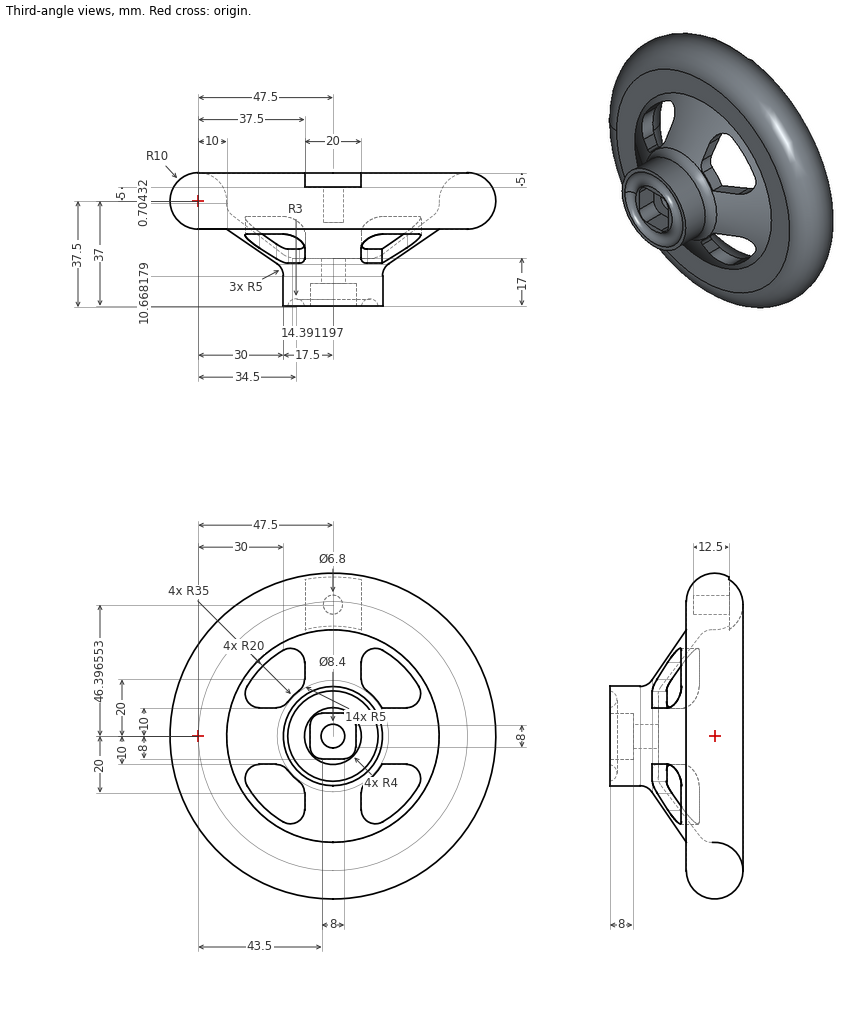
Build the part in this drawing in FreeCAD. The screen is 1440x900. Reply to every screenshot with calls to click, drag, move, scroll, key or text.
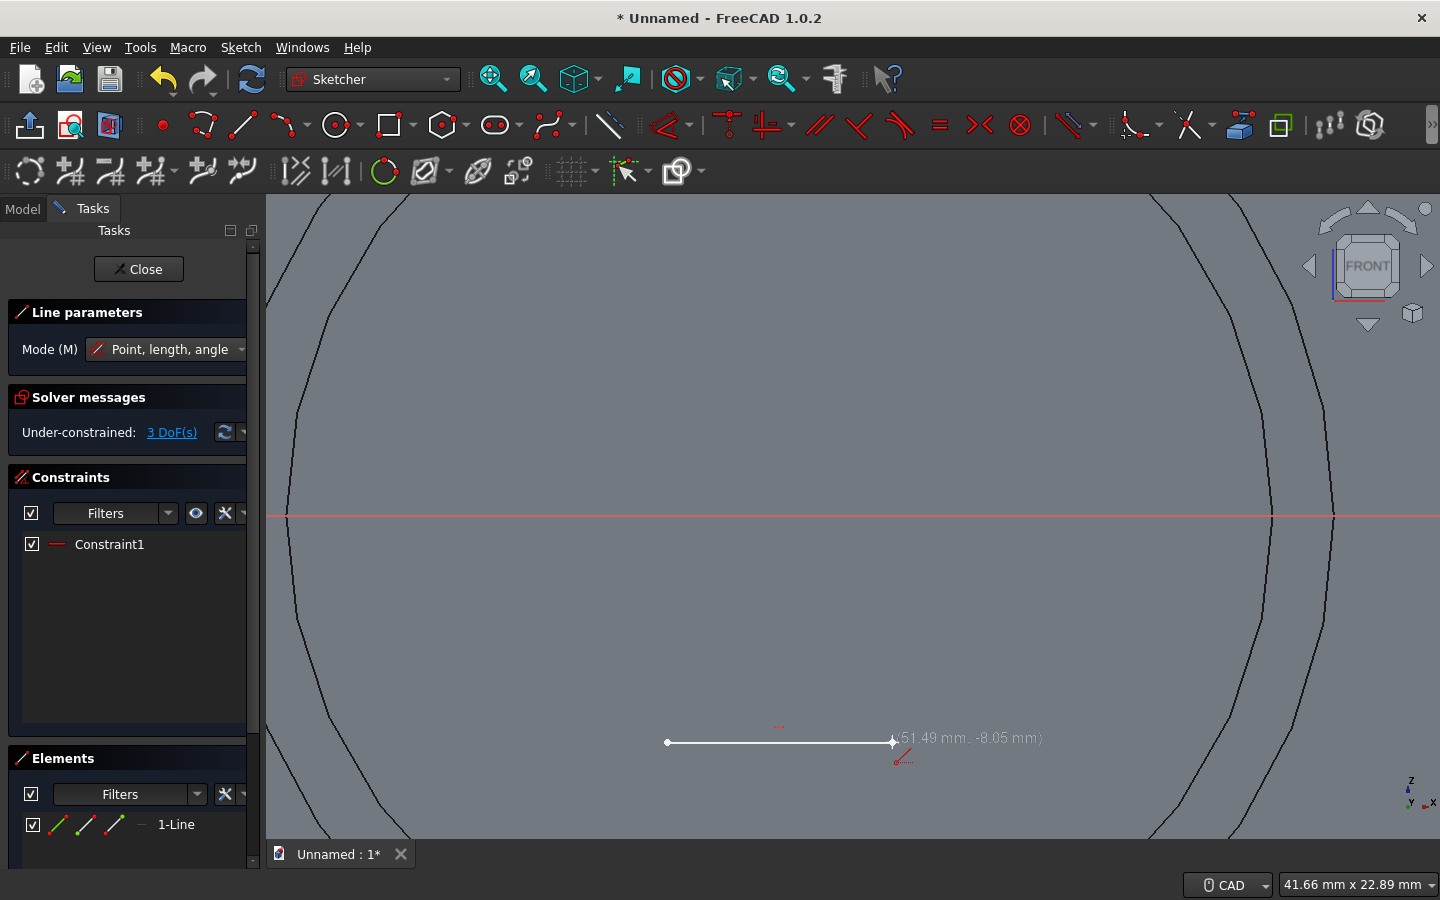
click(1005, 629)
click(1005, 403)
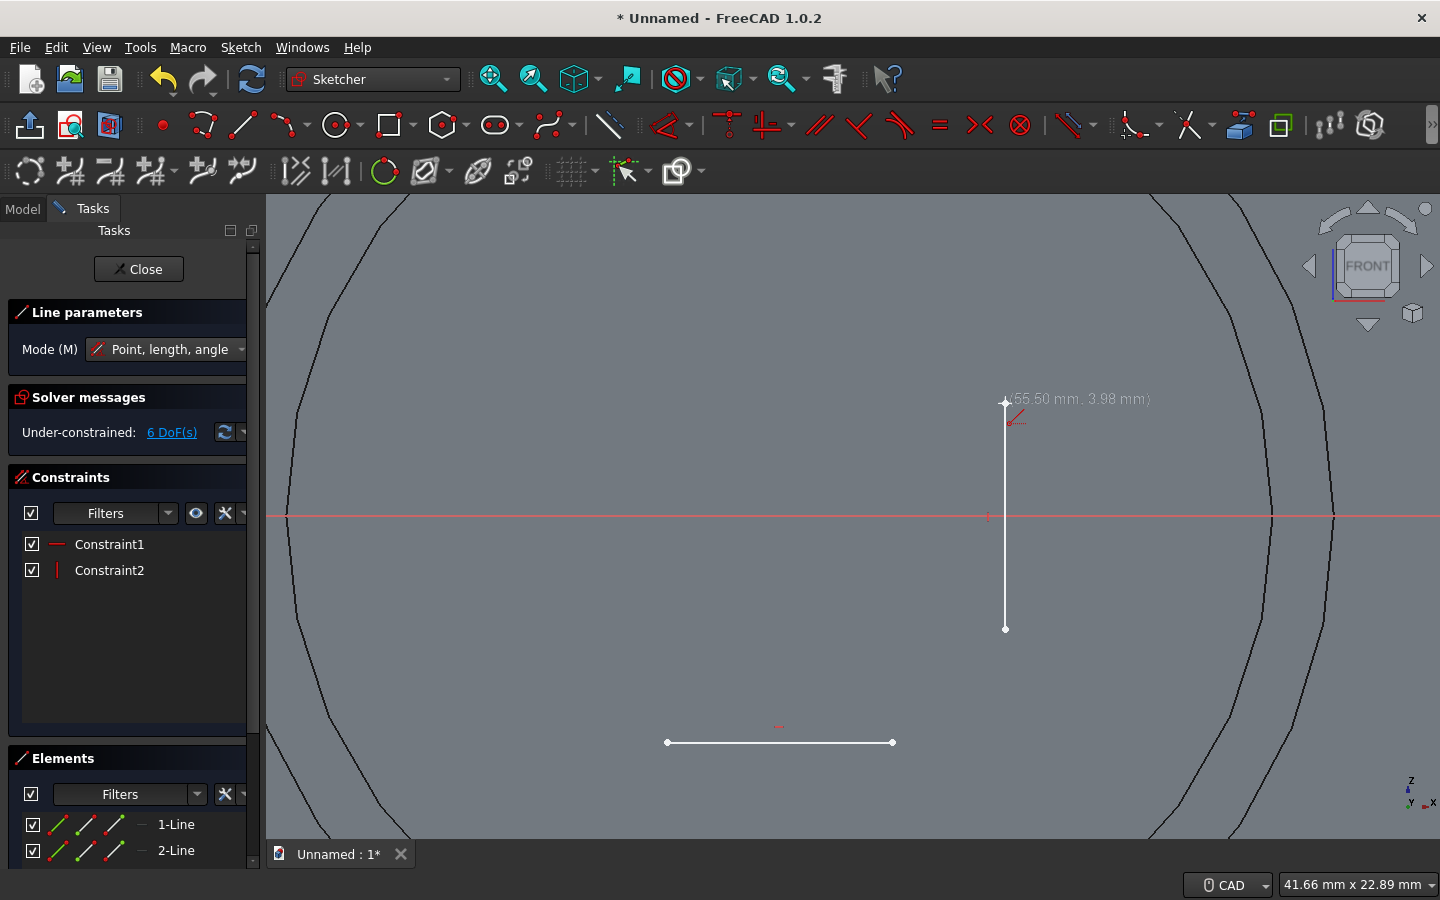
click(892, 291)
click(667, 291)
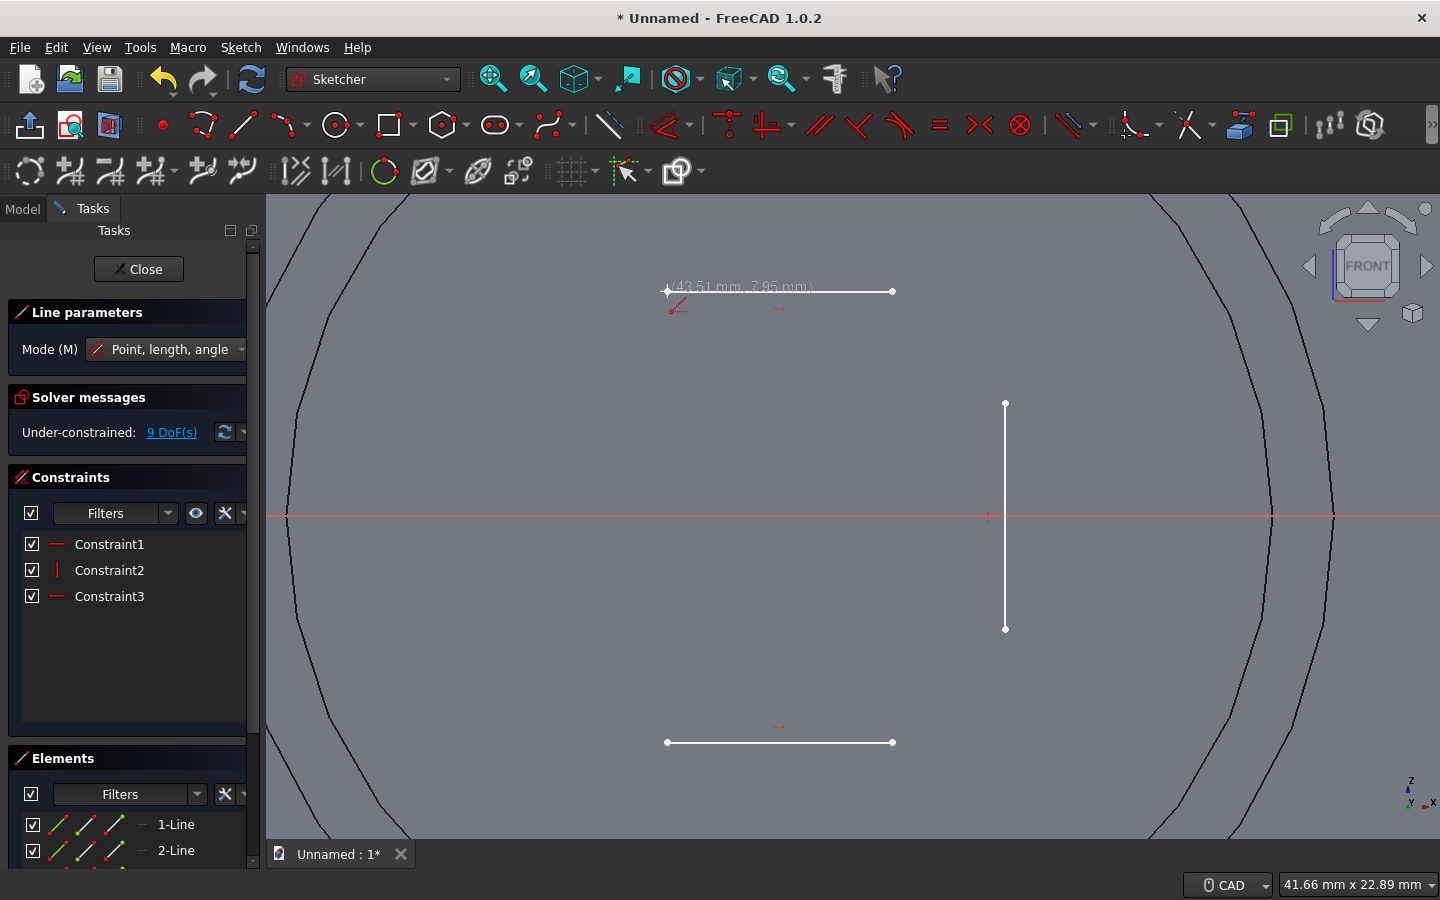
click(554, 403)
click(554, 629)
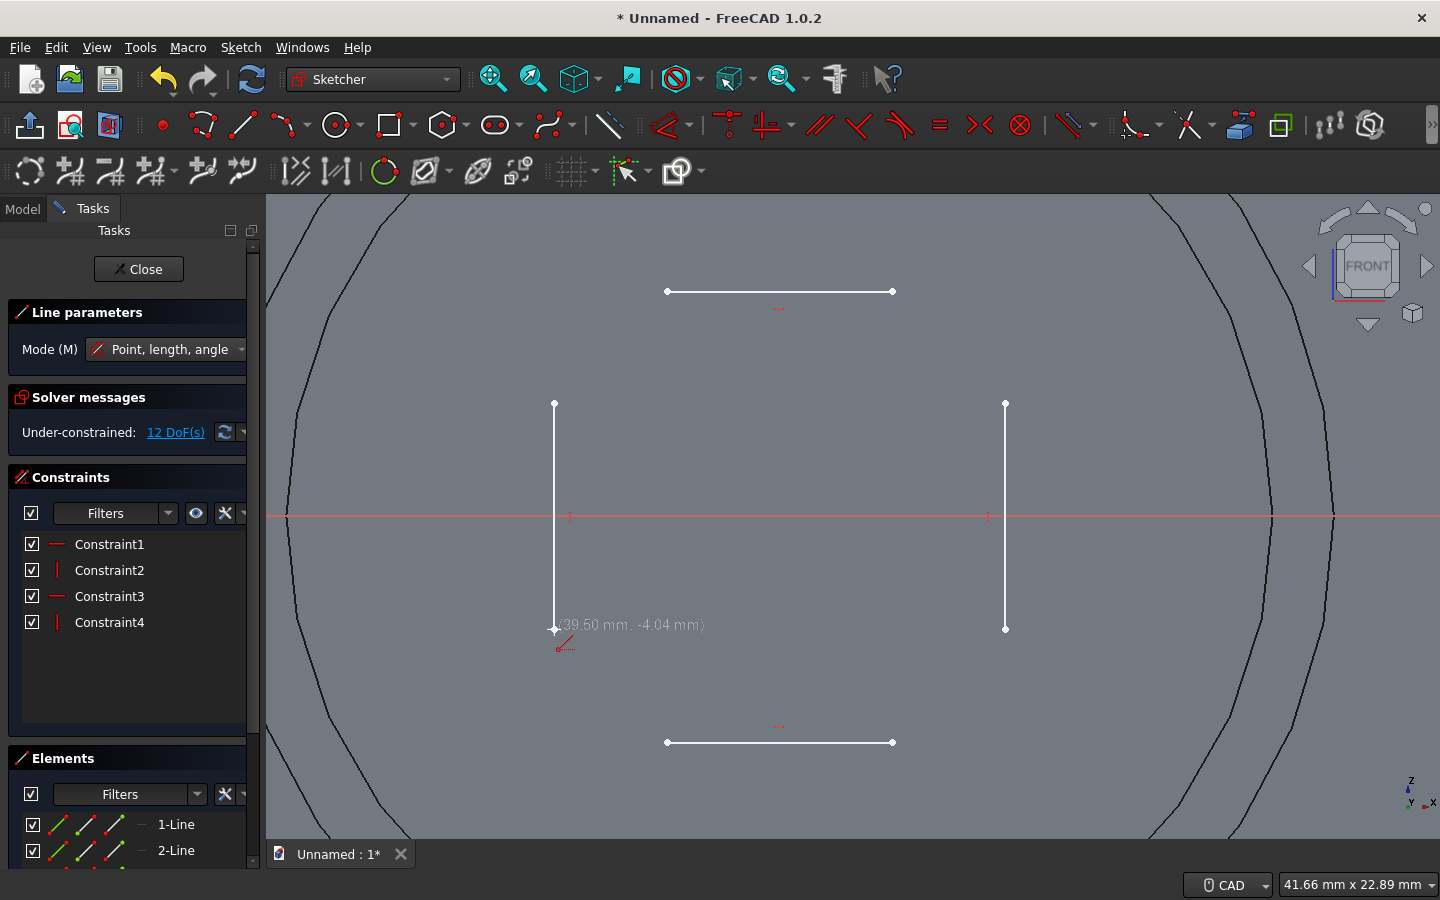
click(284, 126)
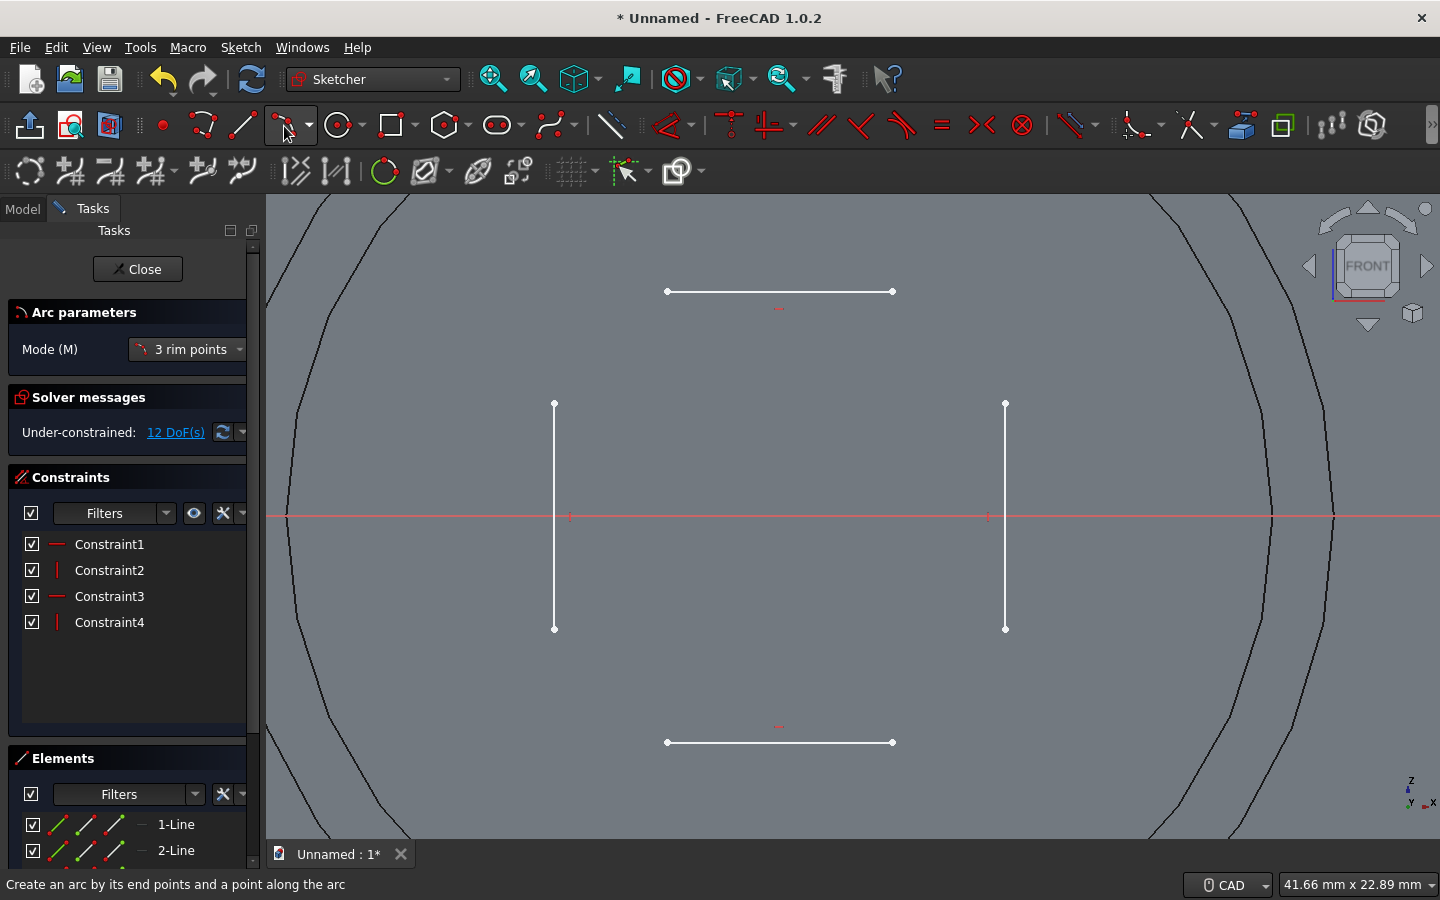
click(892, 743)
click(1005, 630)
click(972, 709)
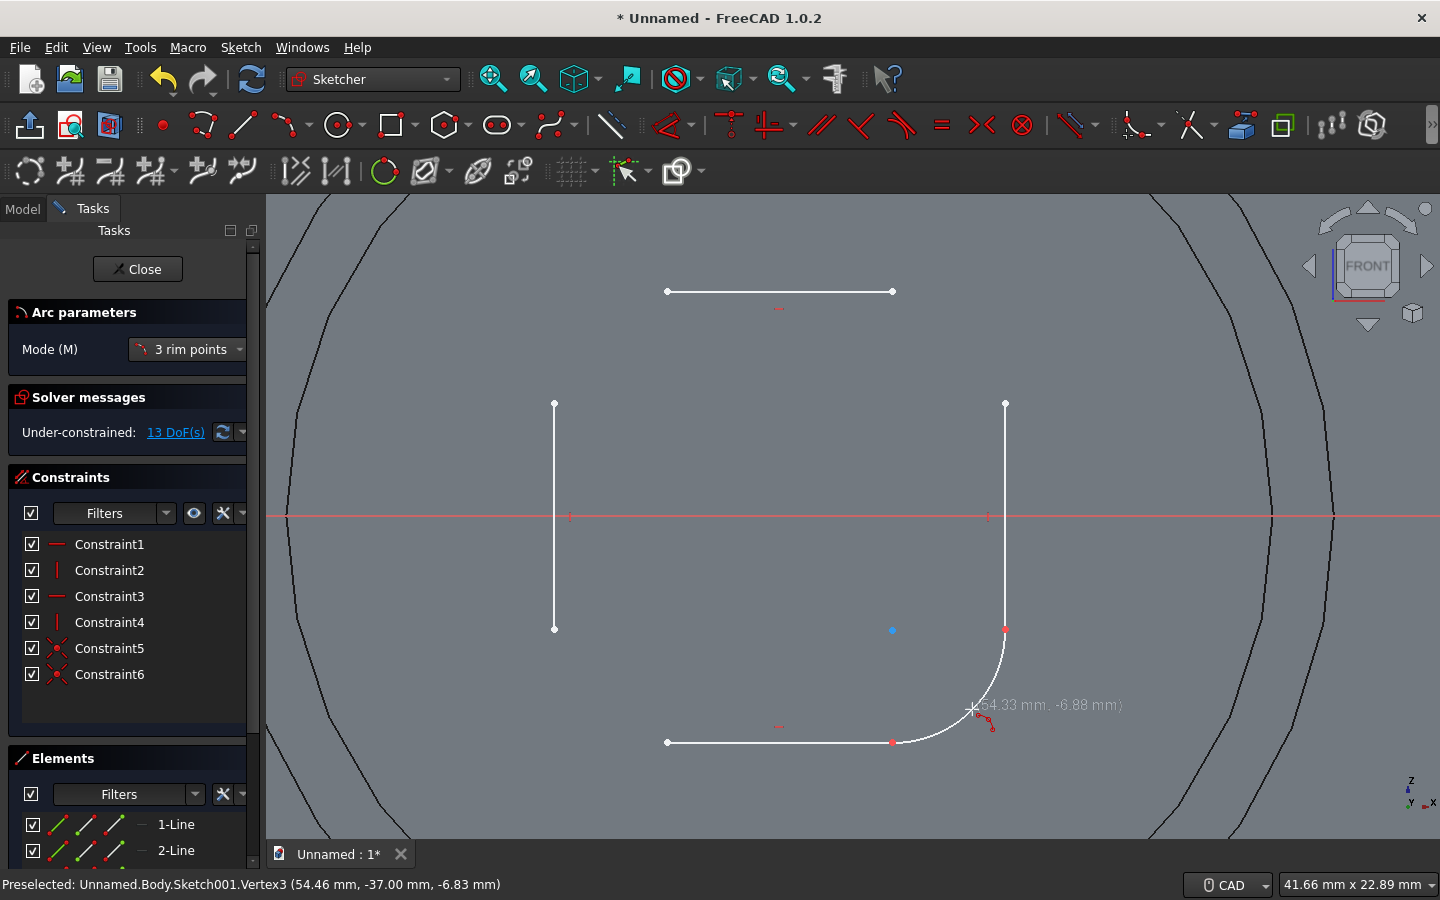
click(1005, 404)
click(892, 292)
click(972, 324)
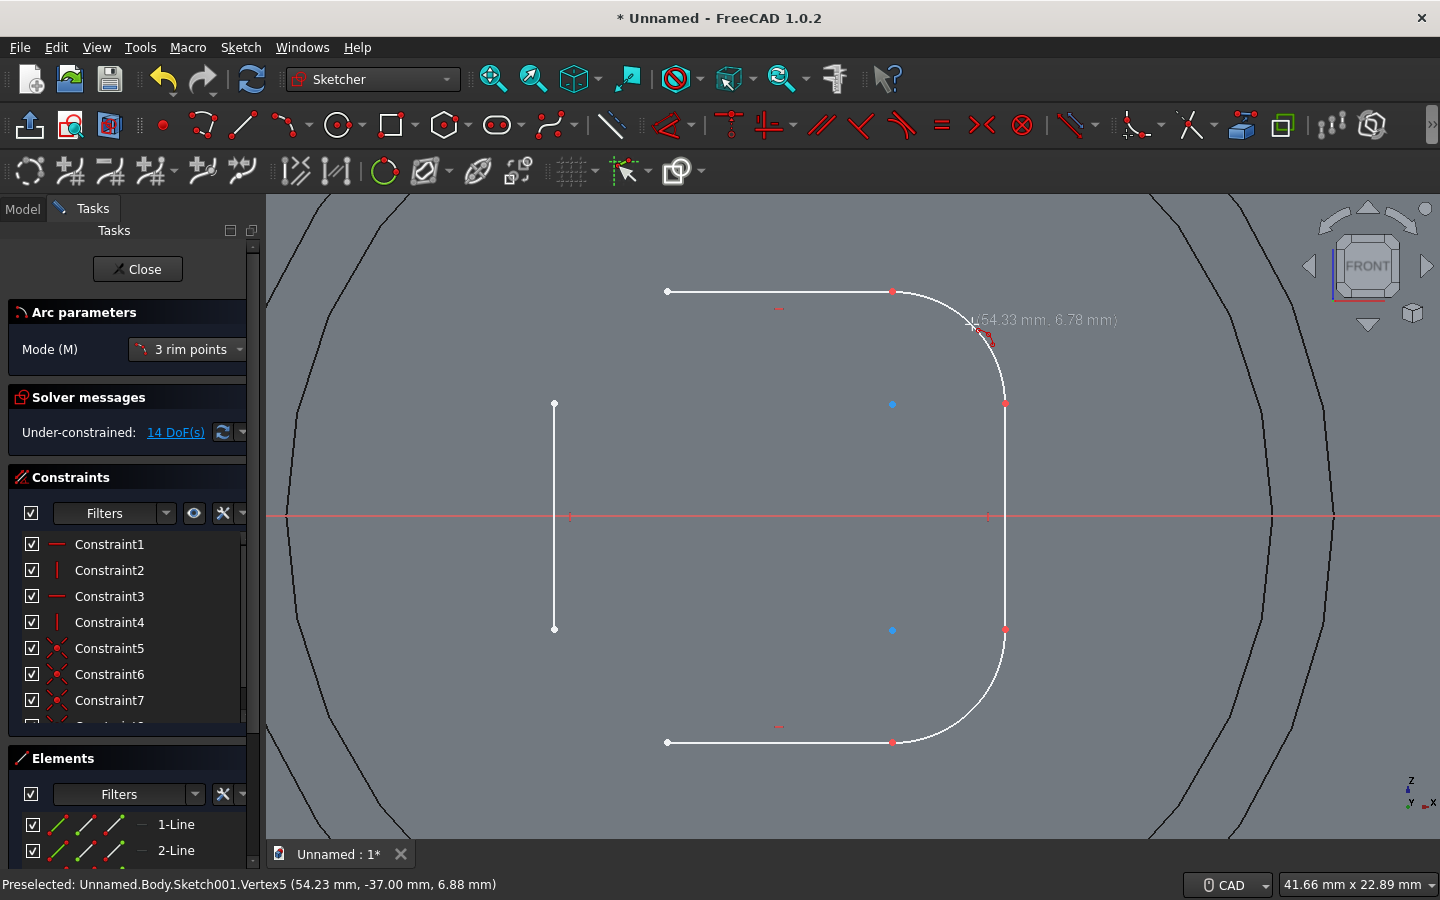
click(667, 292)
click(554, 404)
click(587, 324)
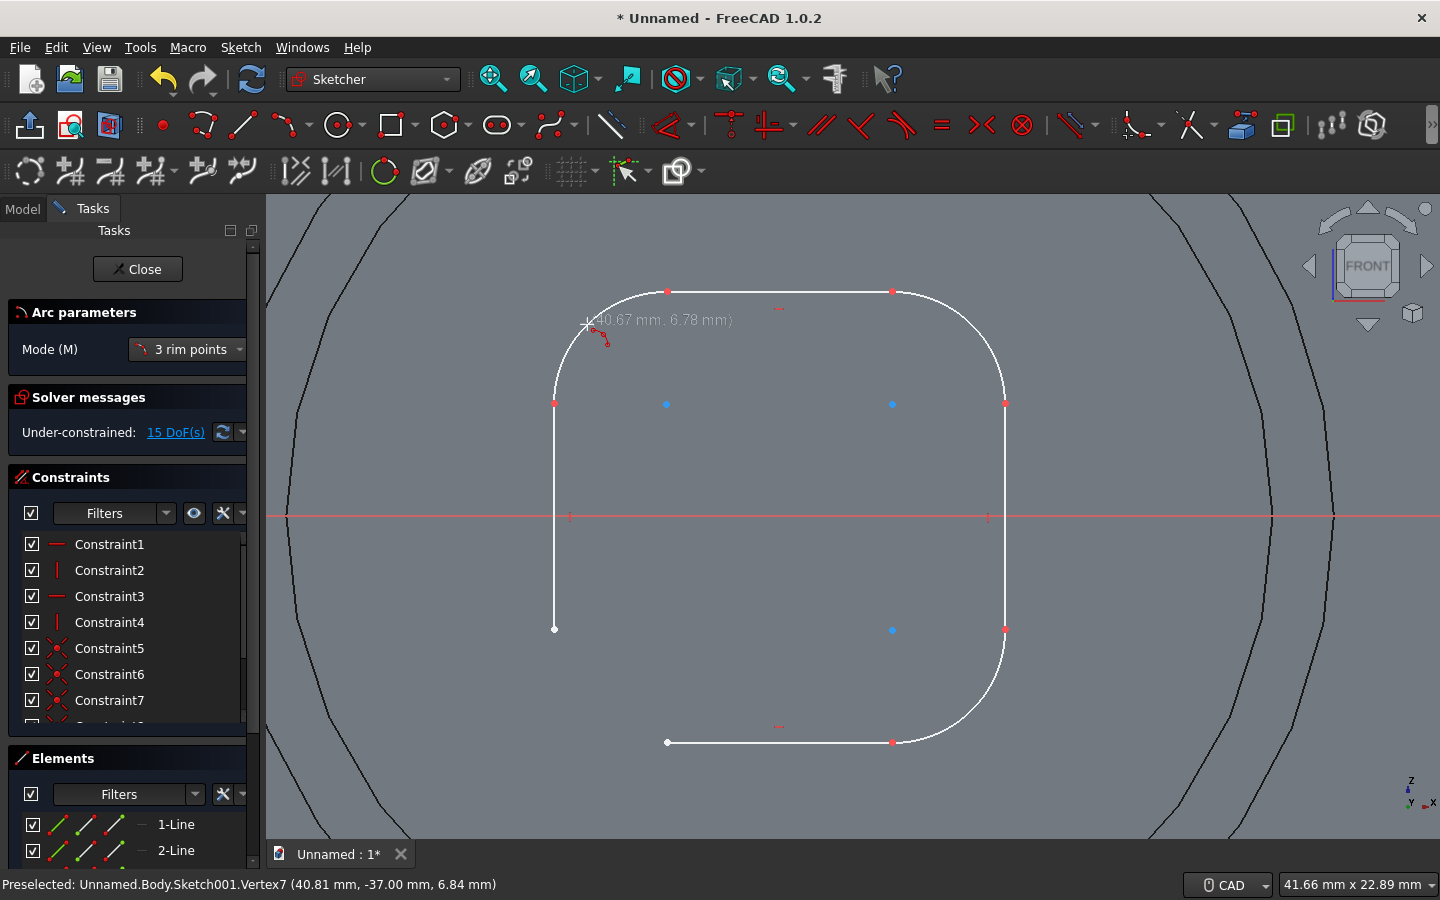
click(554, 630)
click(667, 743)
click(587, 709)
key(Escape)